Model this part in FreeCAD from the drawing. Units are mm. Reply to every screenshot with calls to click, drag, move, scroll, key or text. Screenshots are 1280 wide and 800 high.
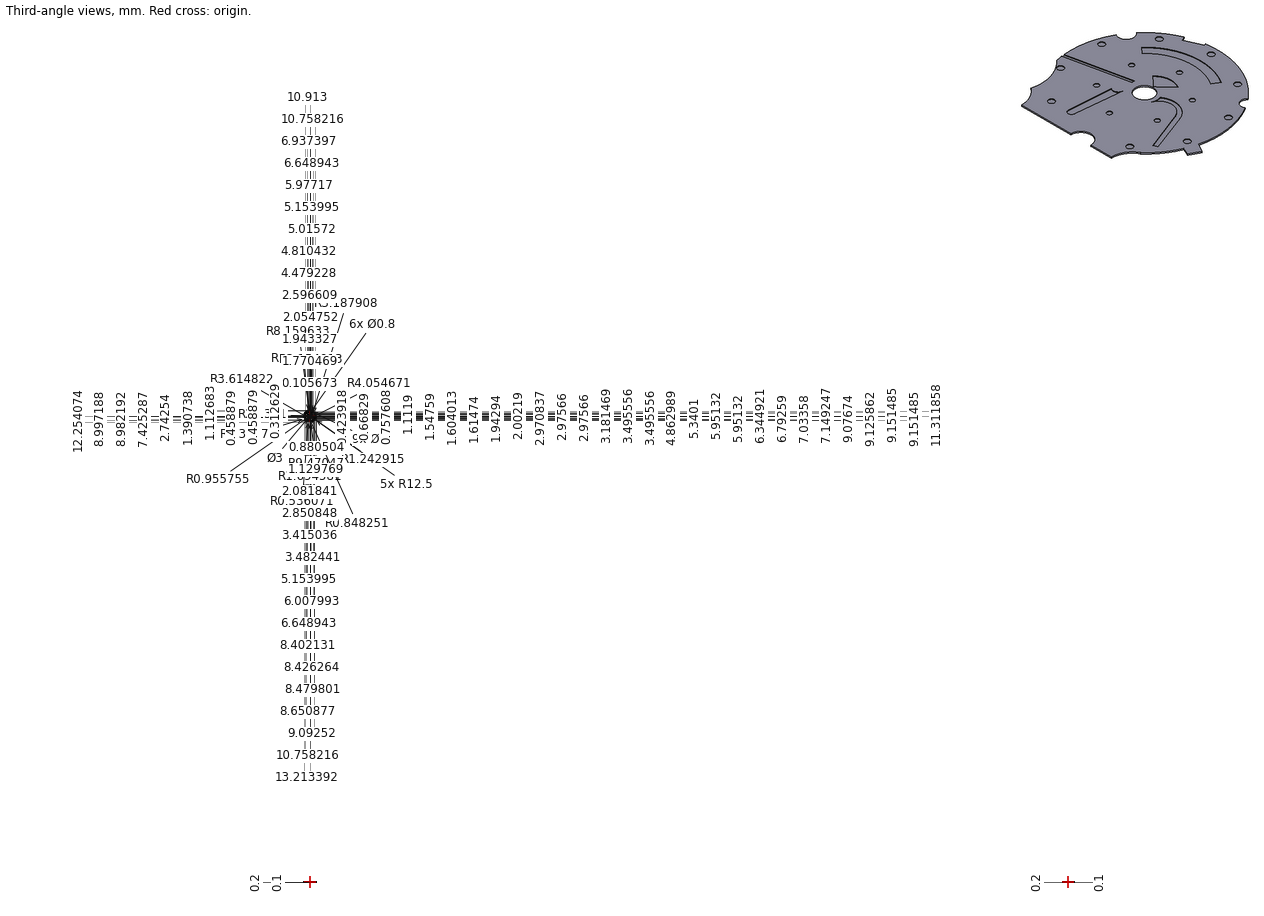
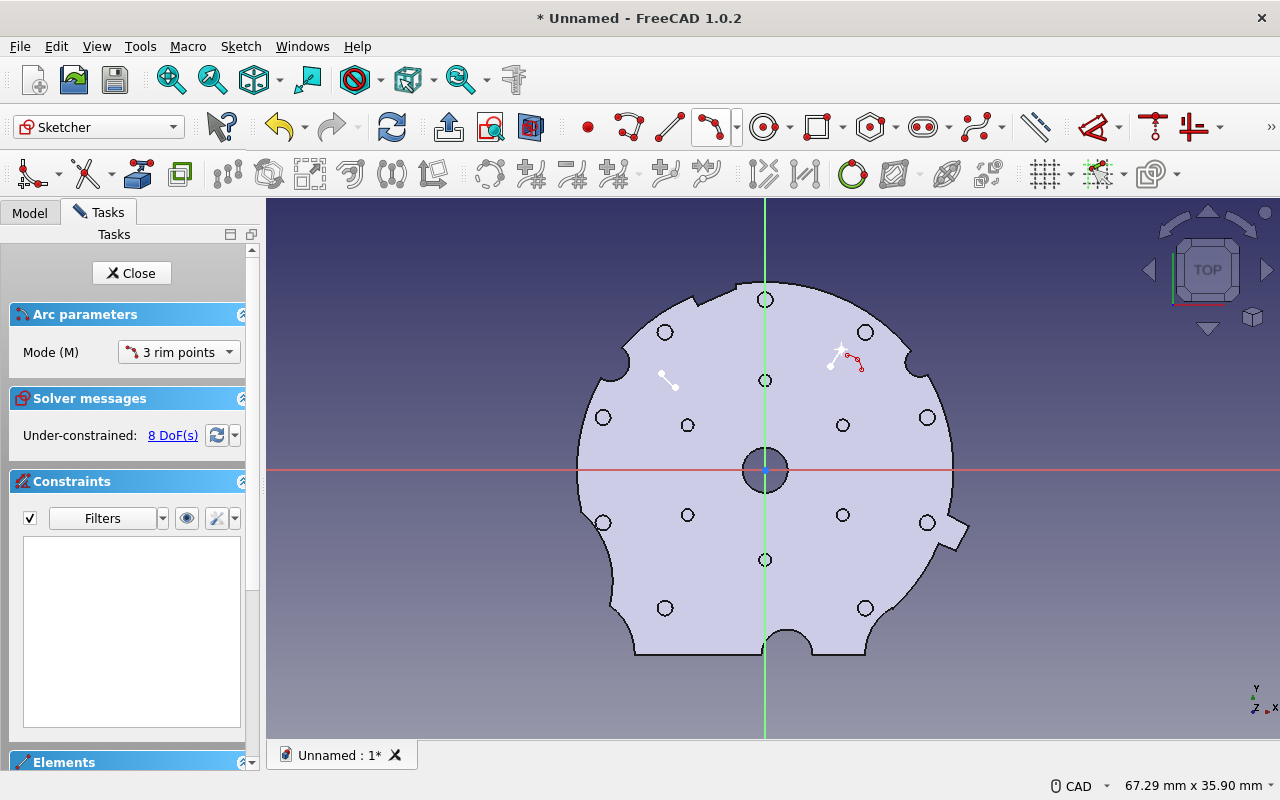
scroll(675, 387, up, 3)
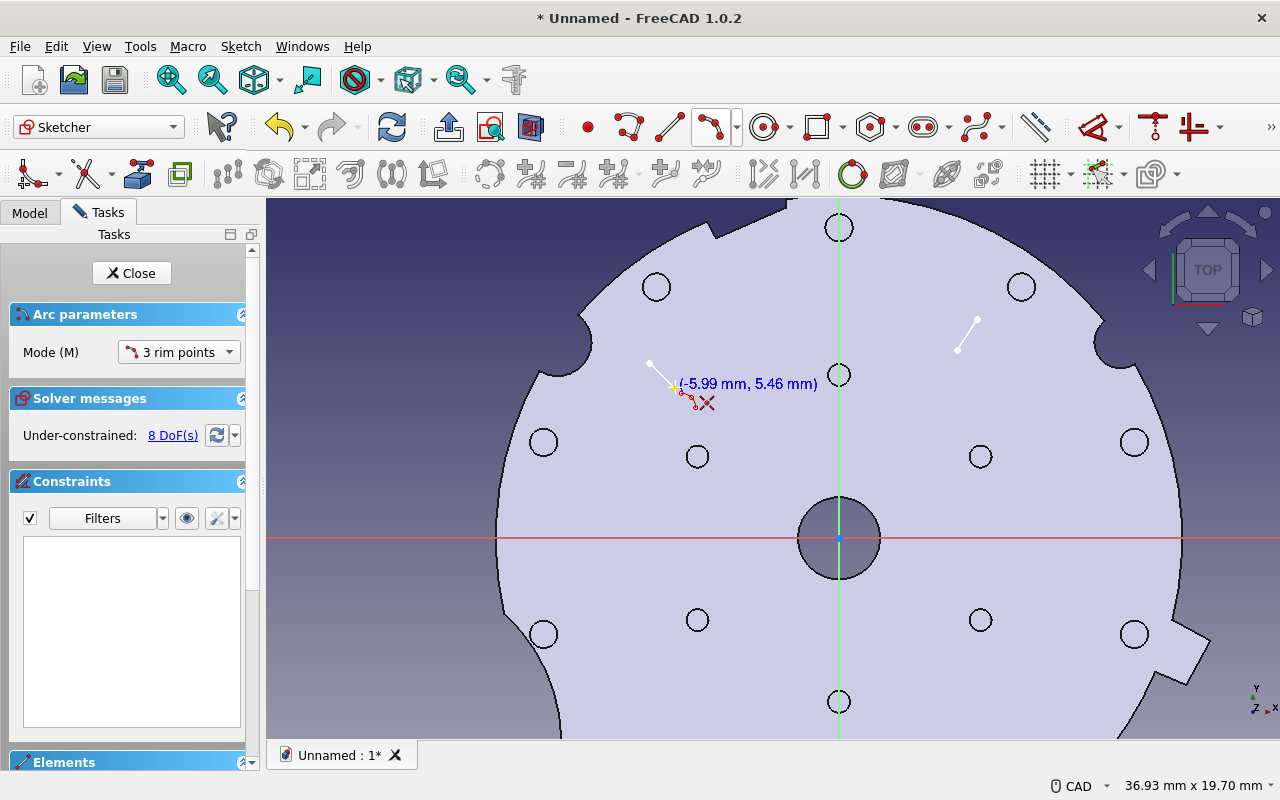
click(675, 389)
click(957, 350)
click(810, 316)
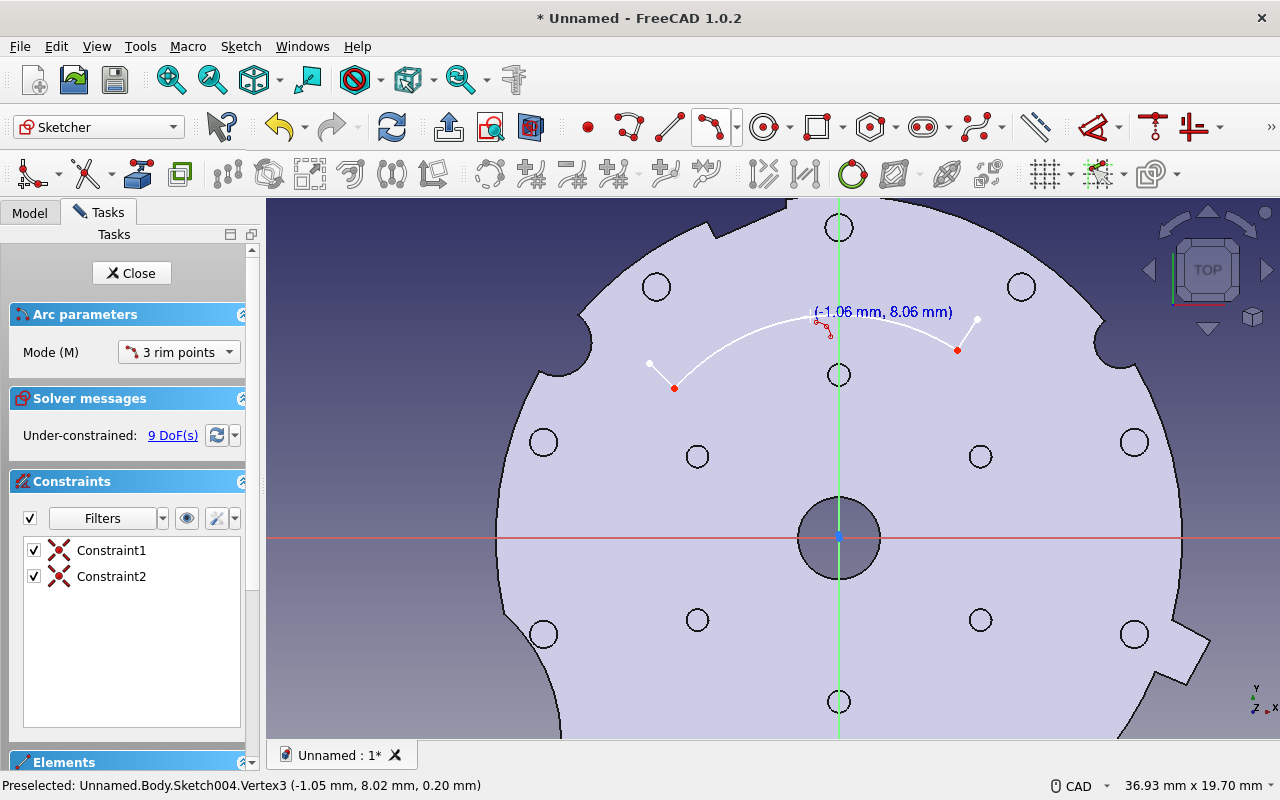
click(977, 319)
click(649, 363)
click(805, 281)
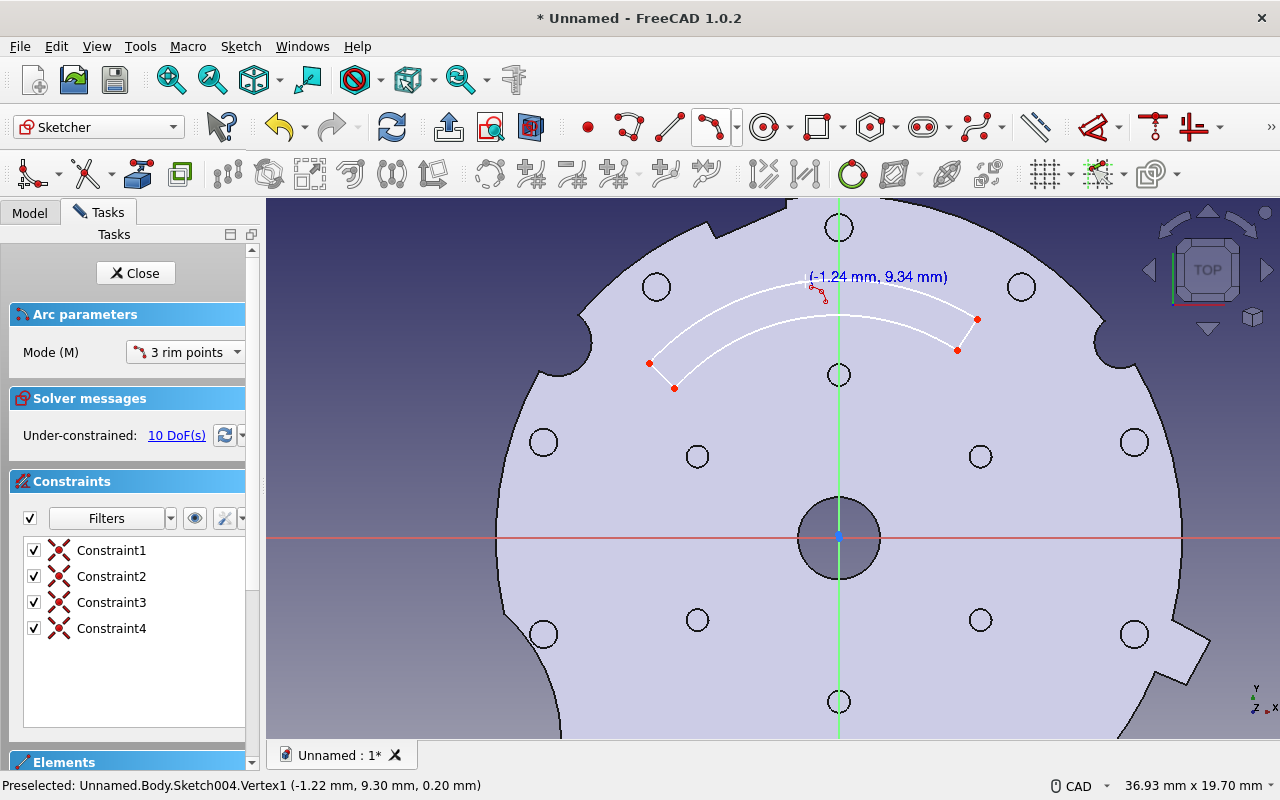
key(g)
key(m)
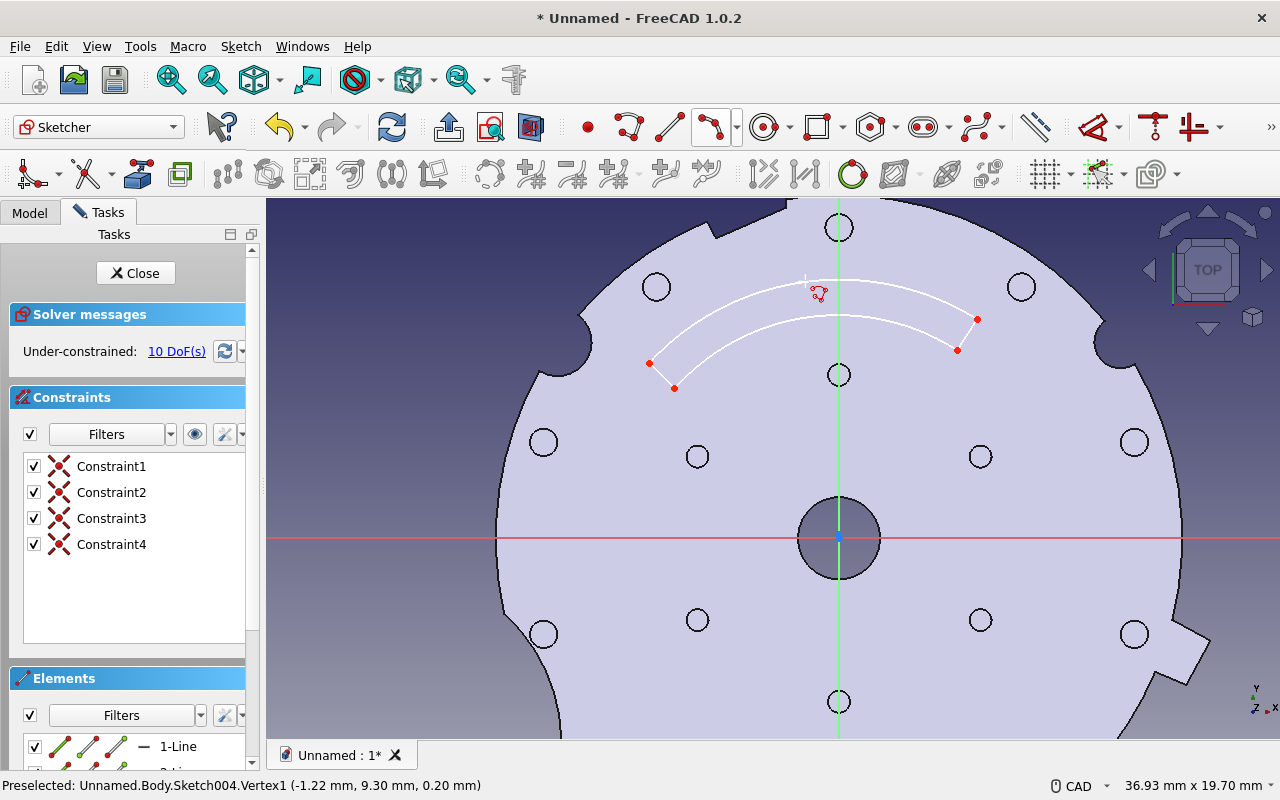
scroll(768, 527, up, 2)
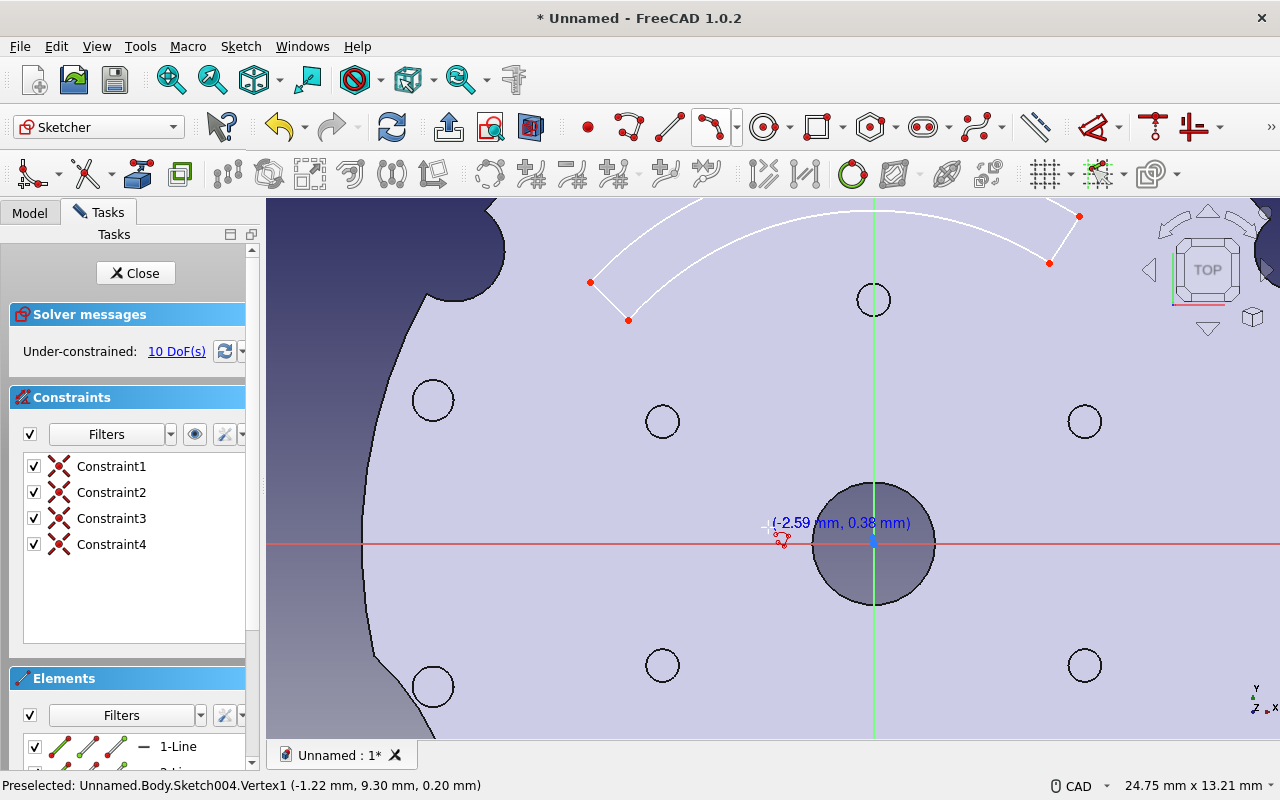
click(767, 526)
click(767, 507)
click(332, 601)
click(332, 619)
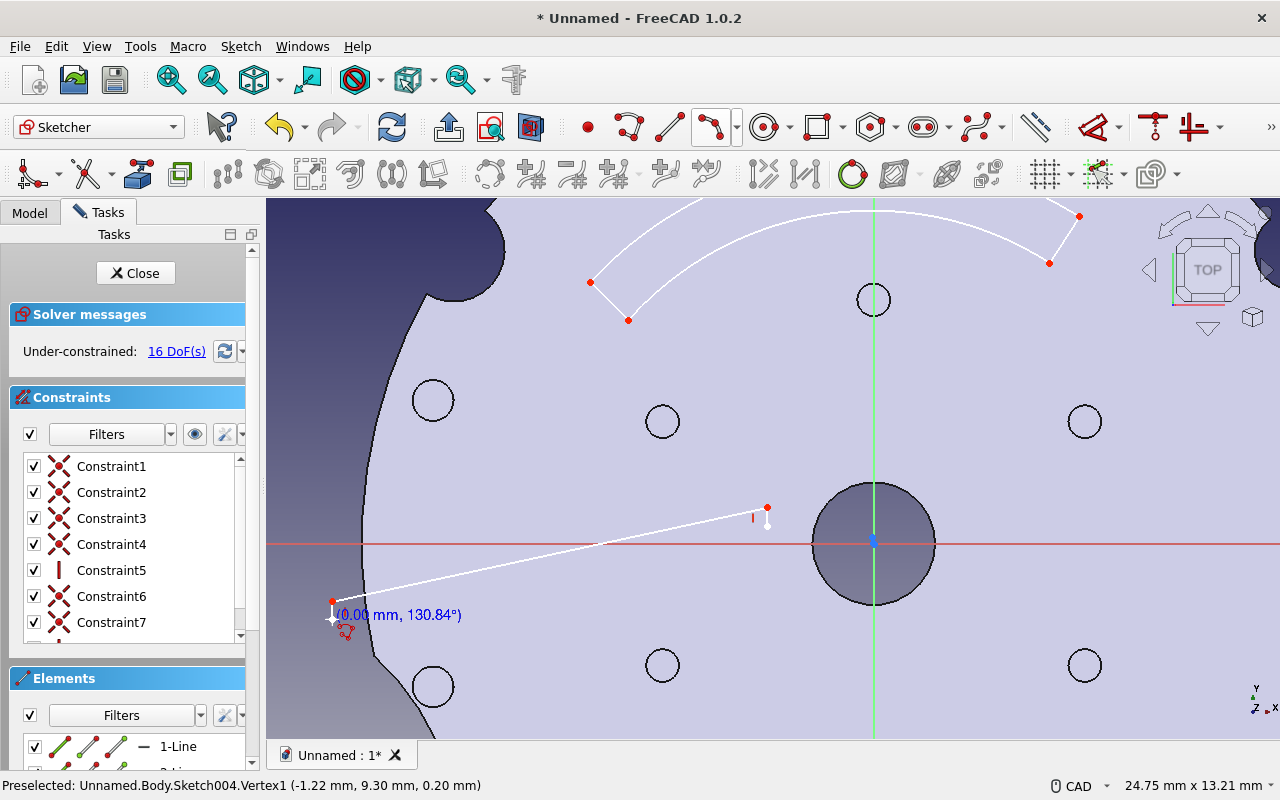
scroll(767, 526, up, 3)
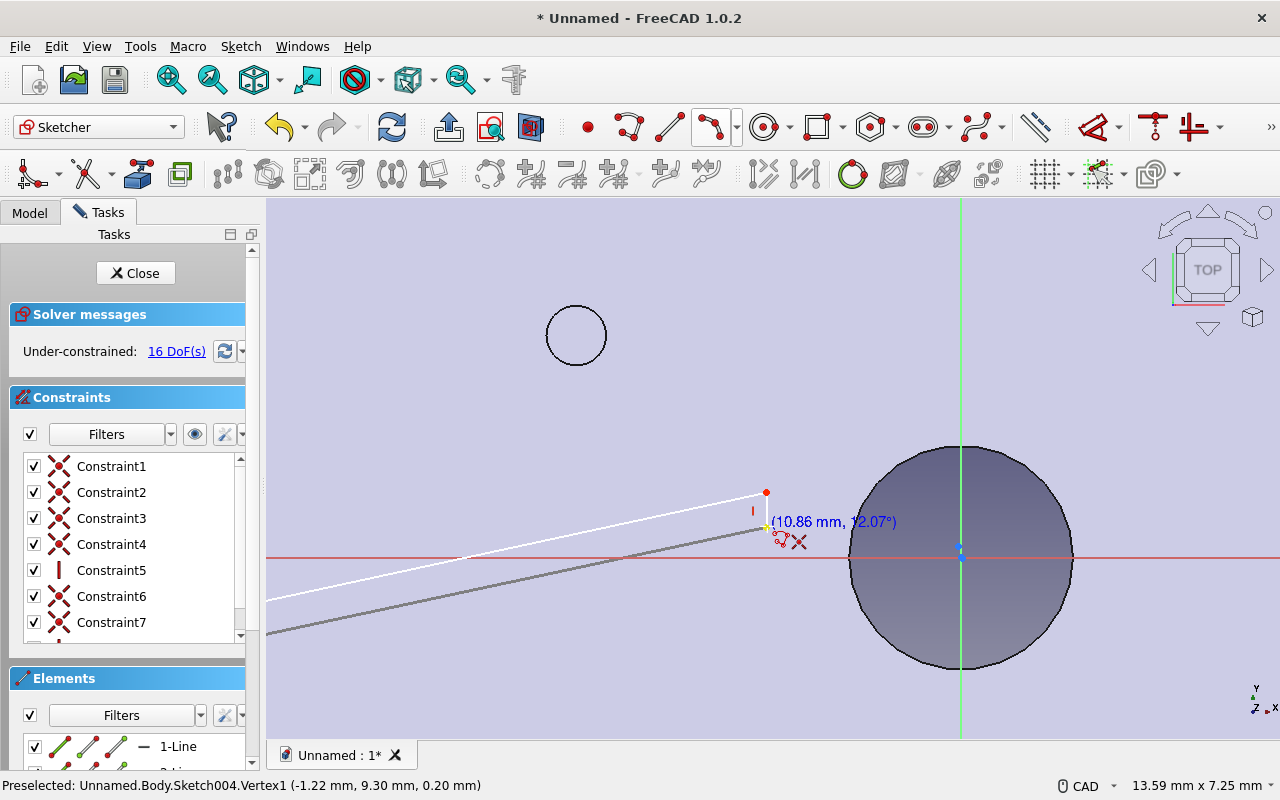
click(767, 527)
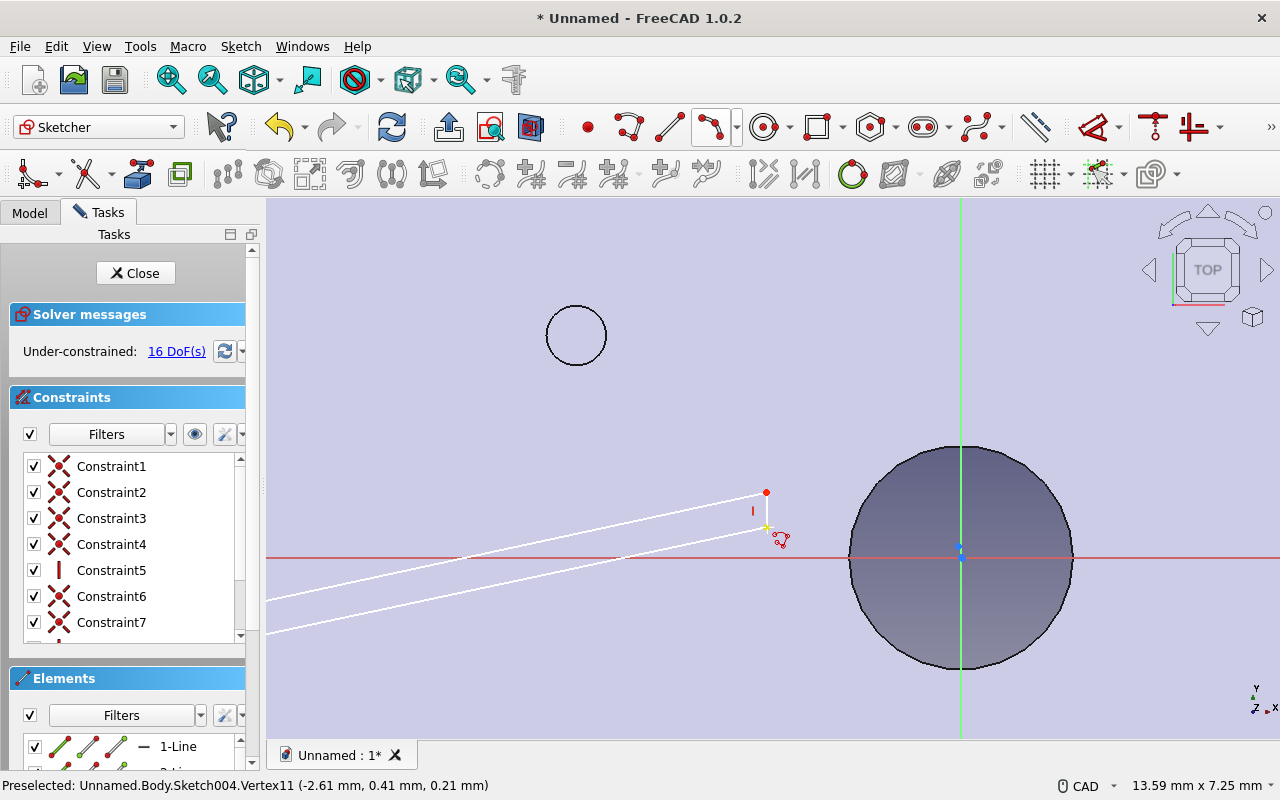
click(670, 128)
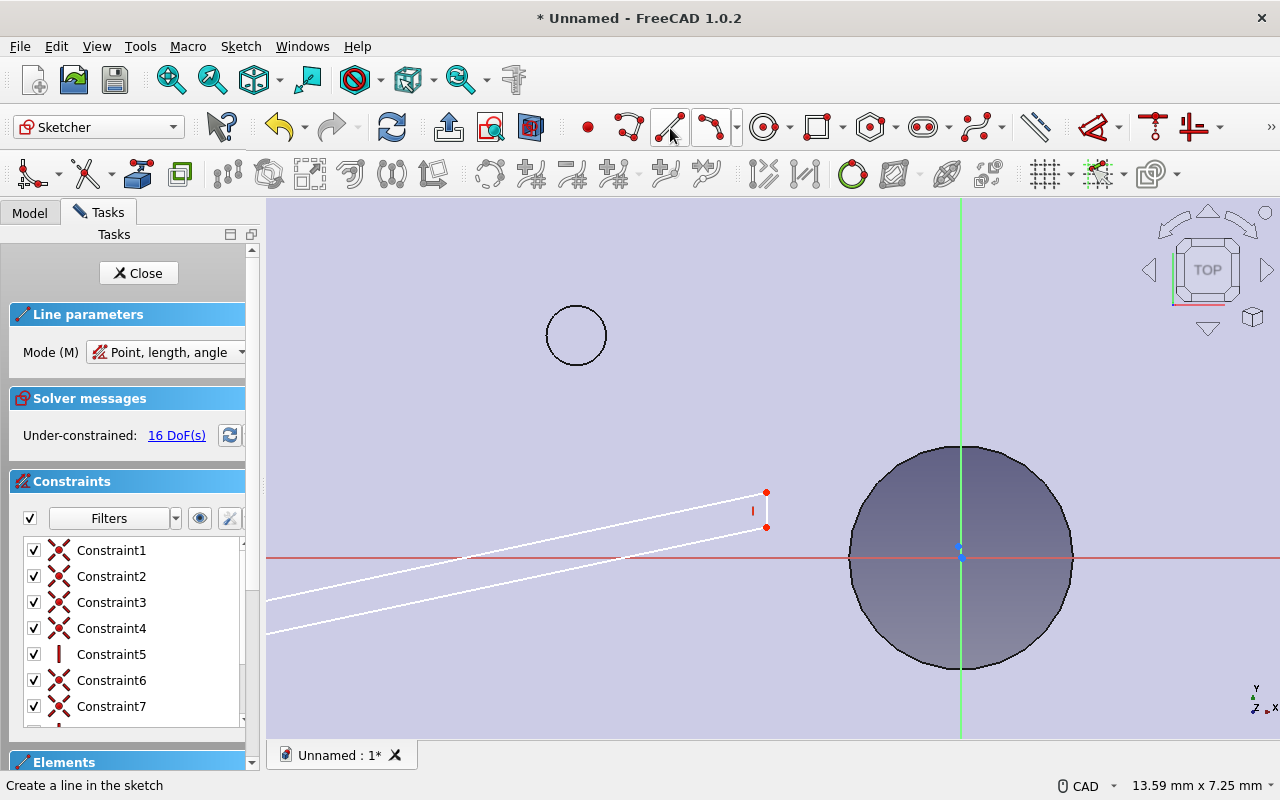
scroll(671, 437, down, 7)